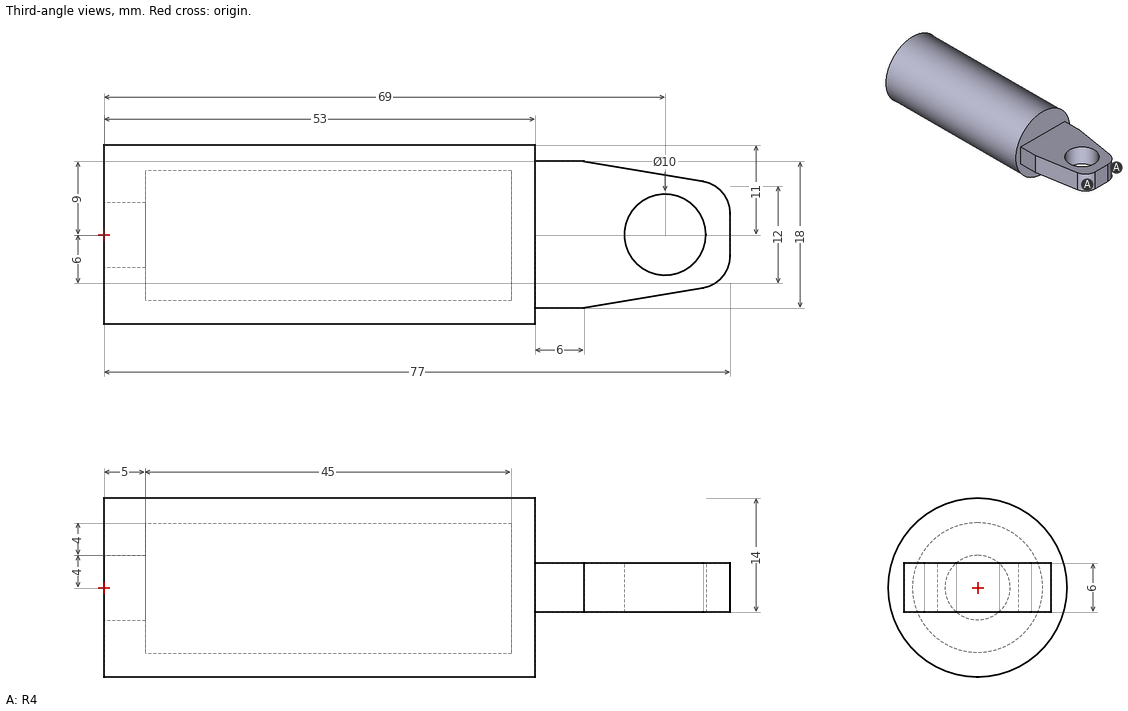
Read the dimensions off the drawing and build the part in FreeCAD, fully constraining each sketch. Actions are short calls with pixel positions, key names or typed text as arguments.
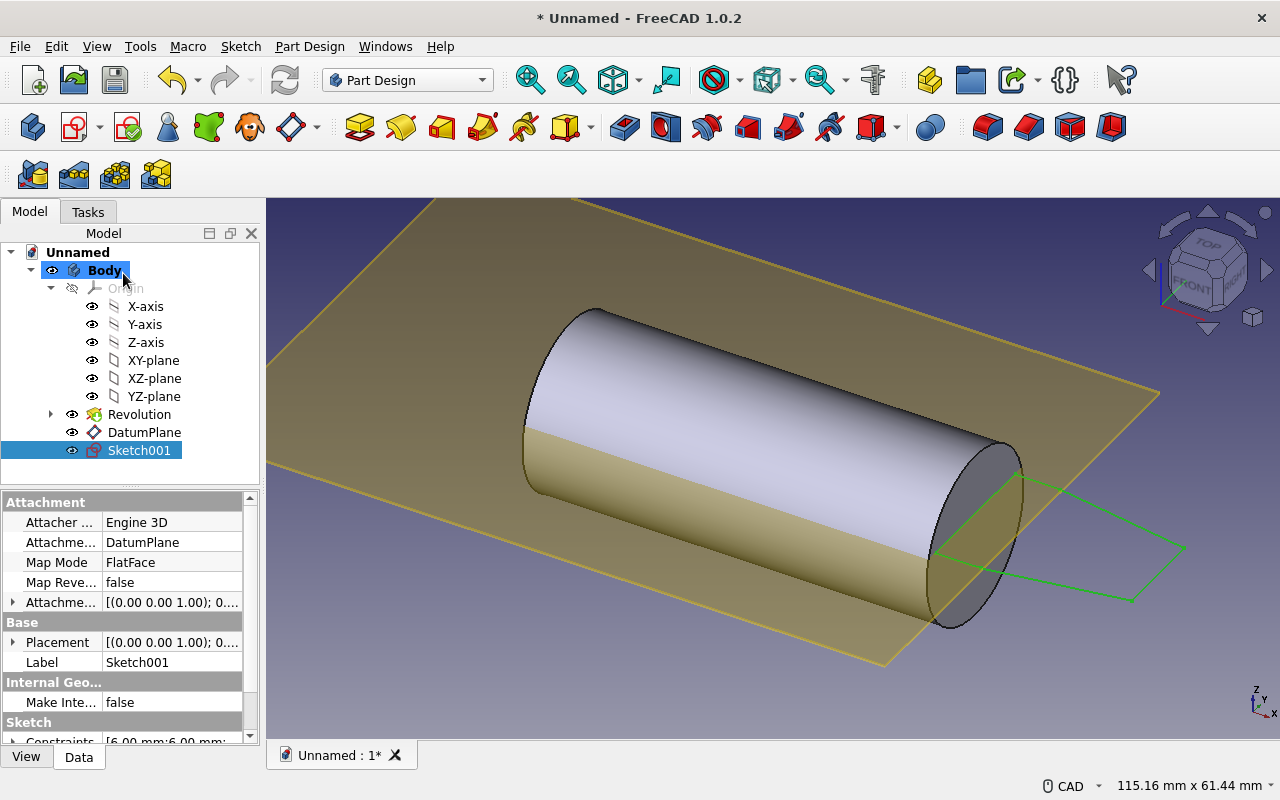
click(360, 128)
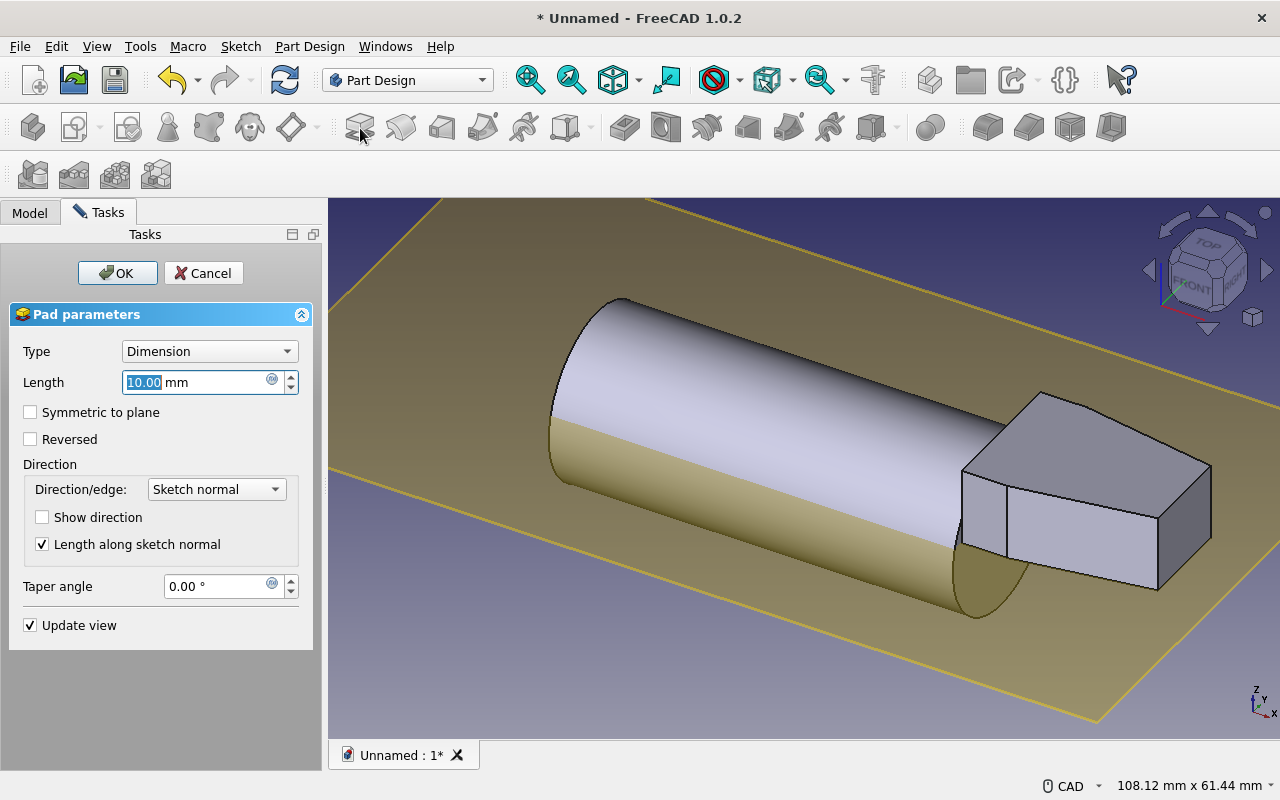
text(6)
key(Tab)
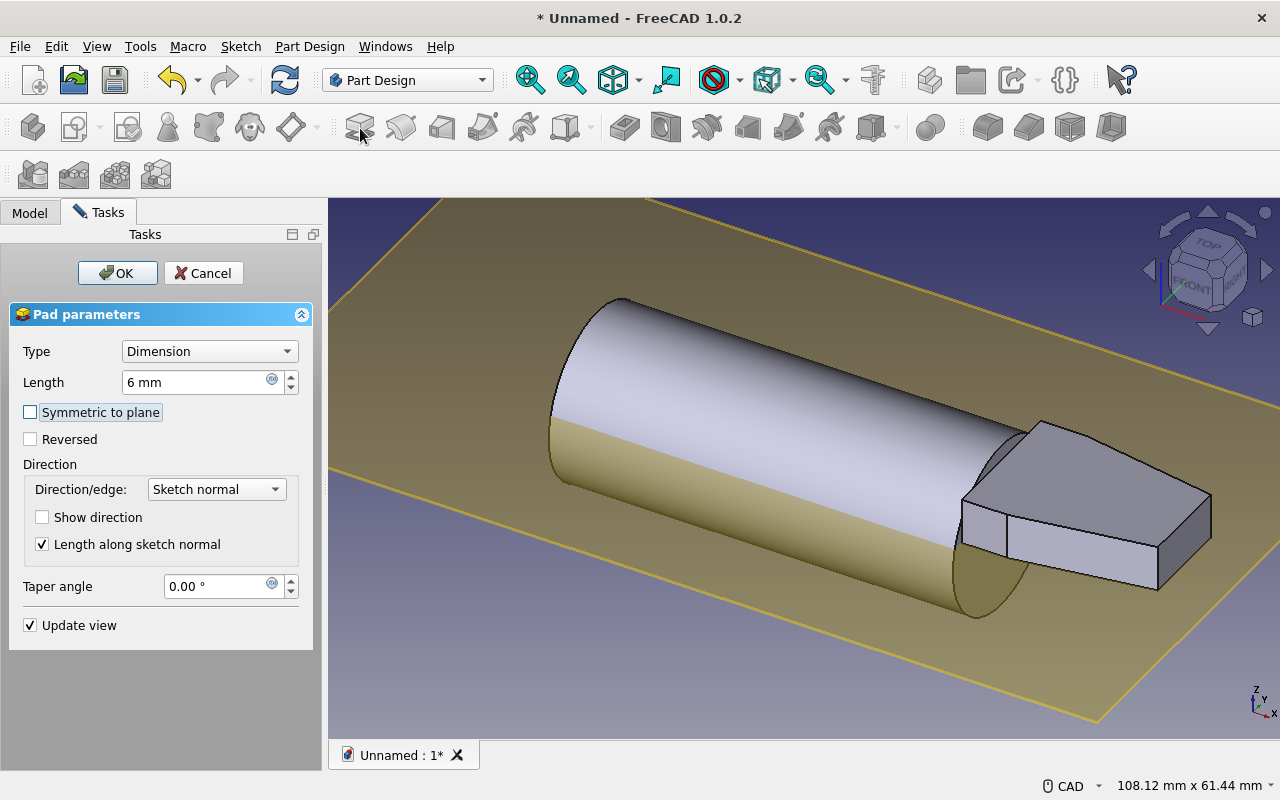
click(31, 439)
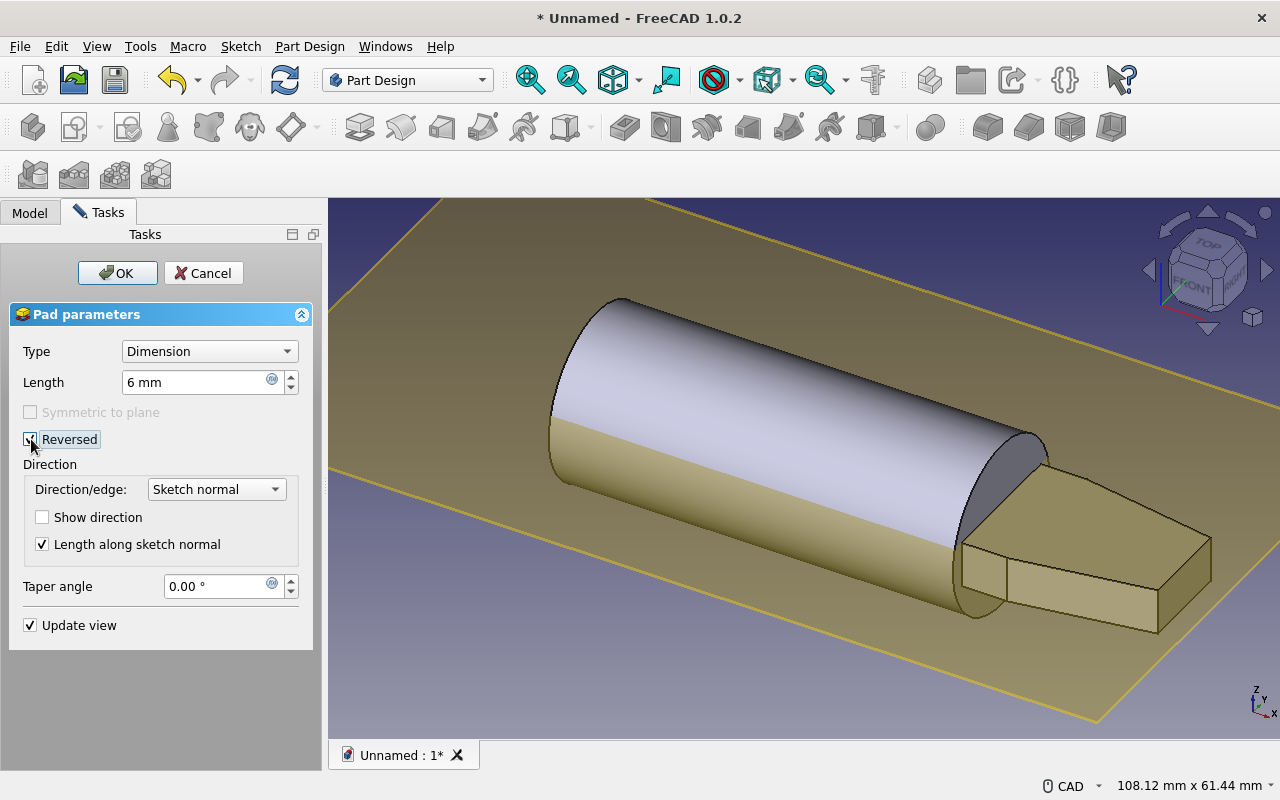
click(118, 273)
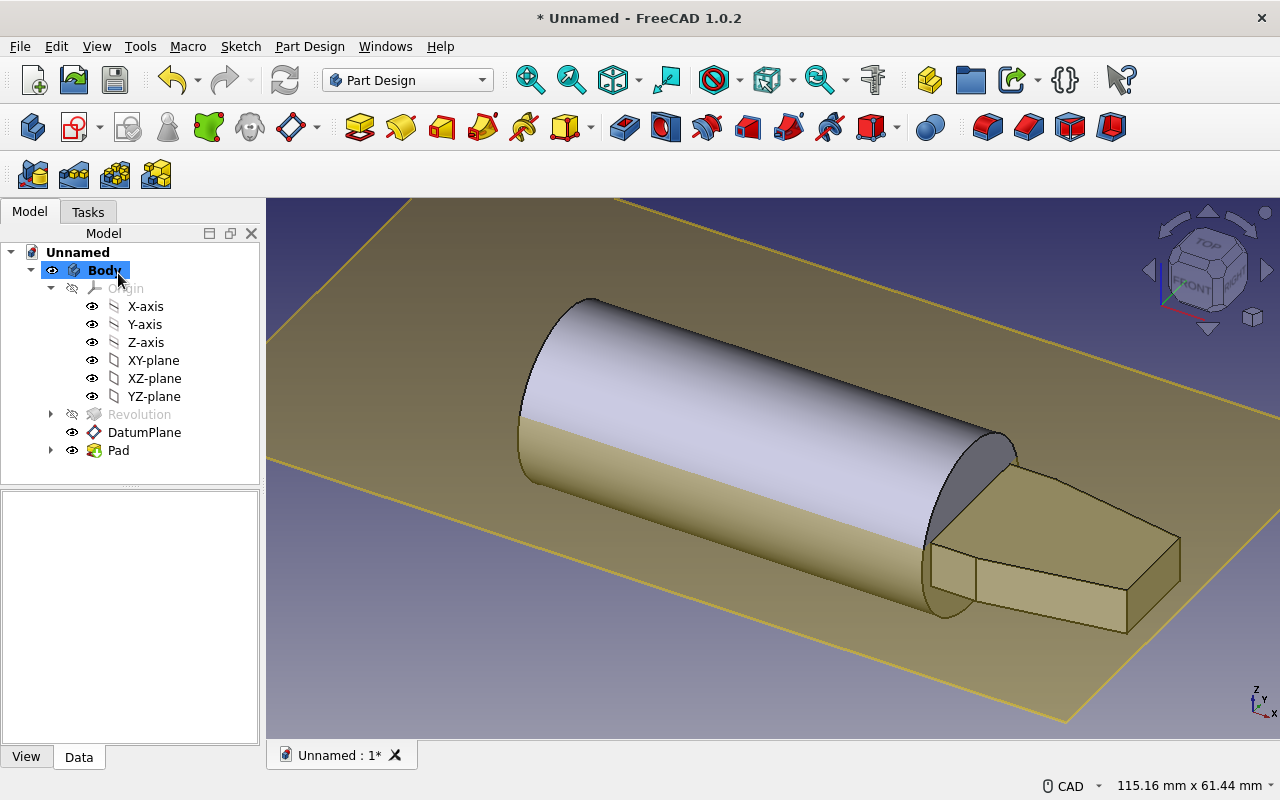
click(117, 432)
key(space)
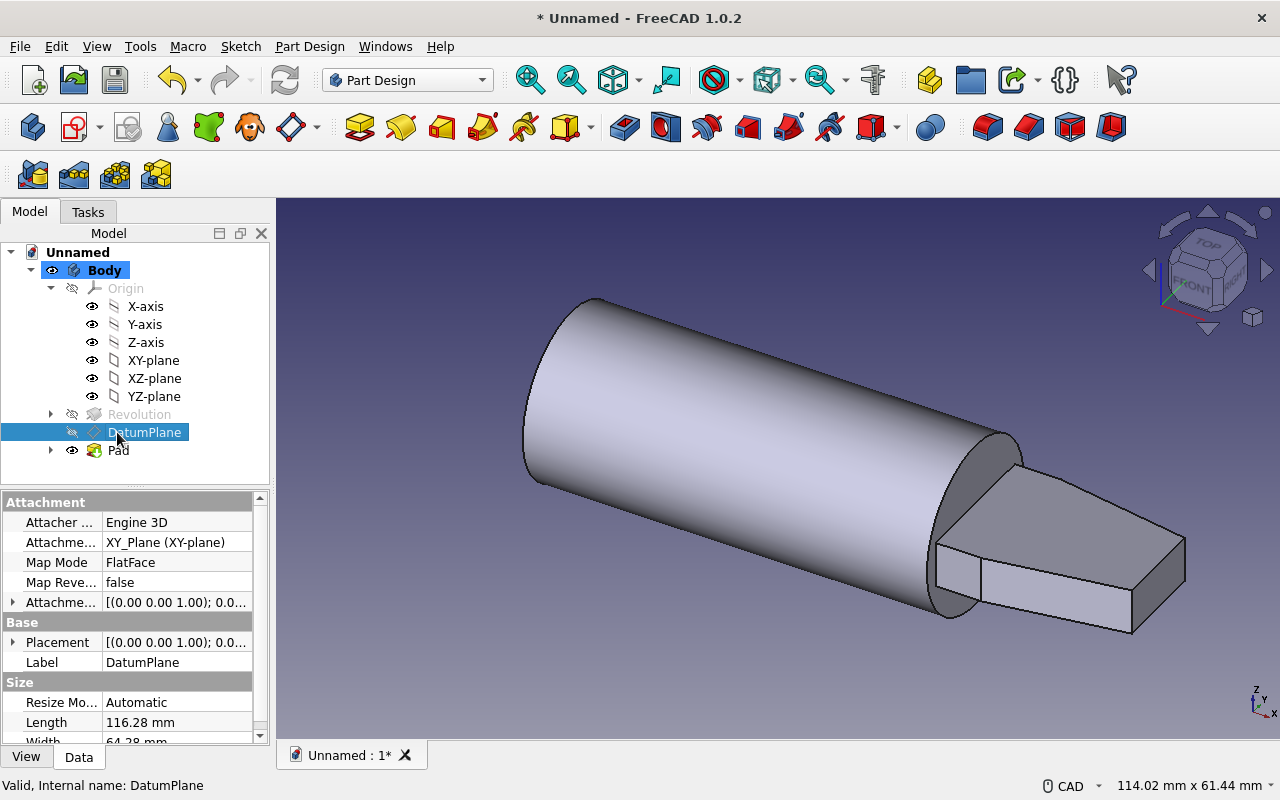
key(5)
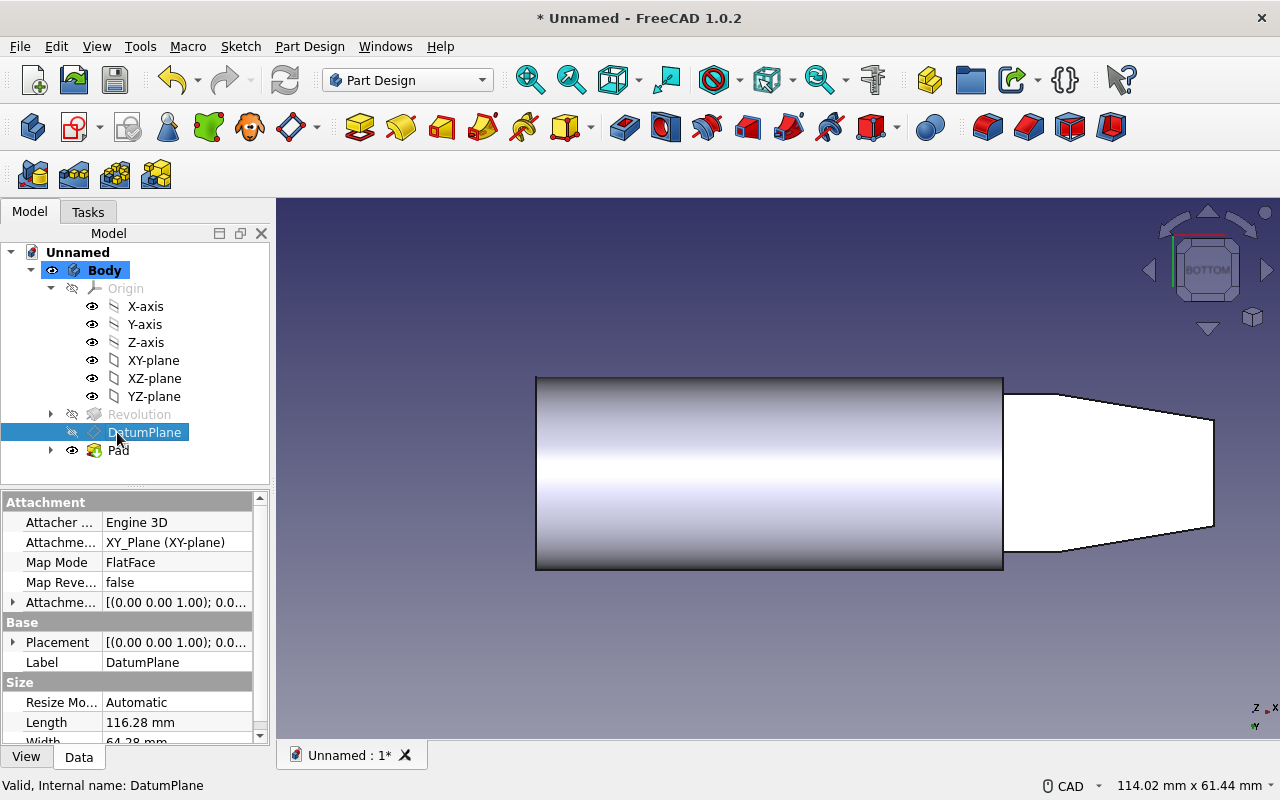
click(1079, 472)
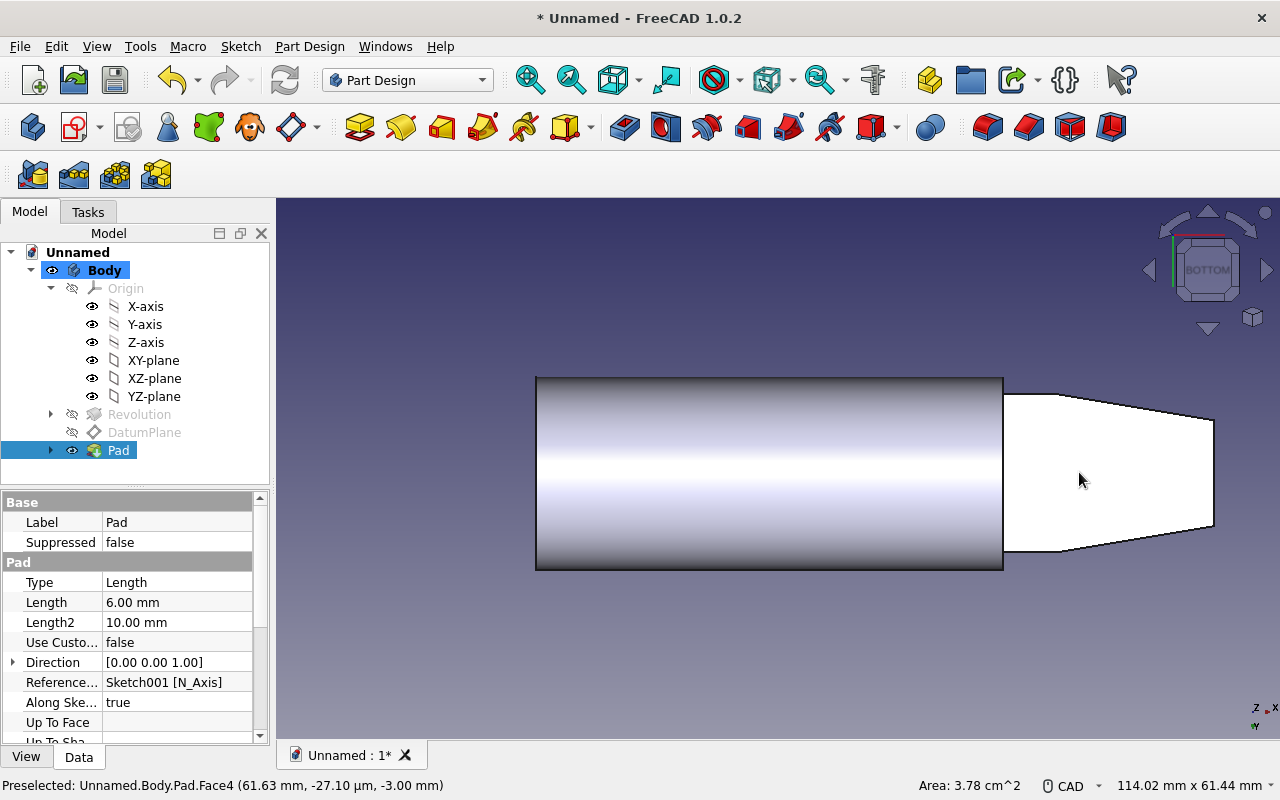
click(74, 128)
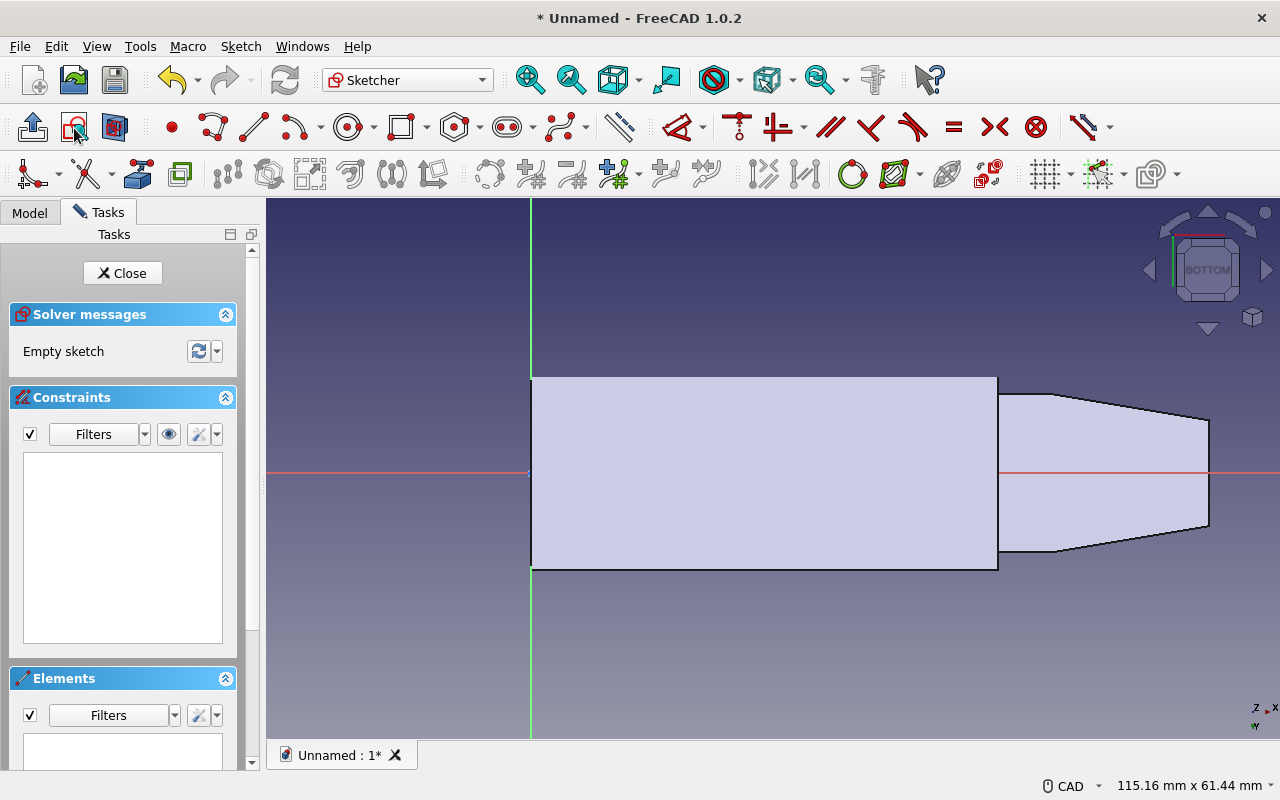
scroll(704, 468, down, 5)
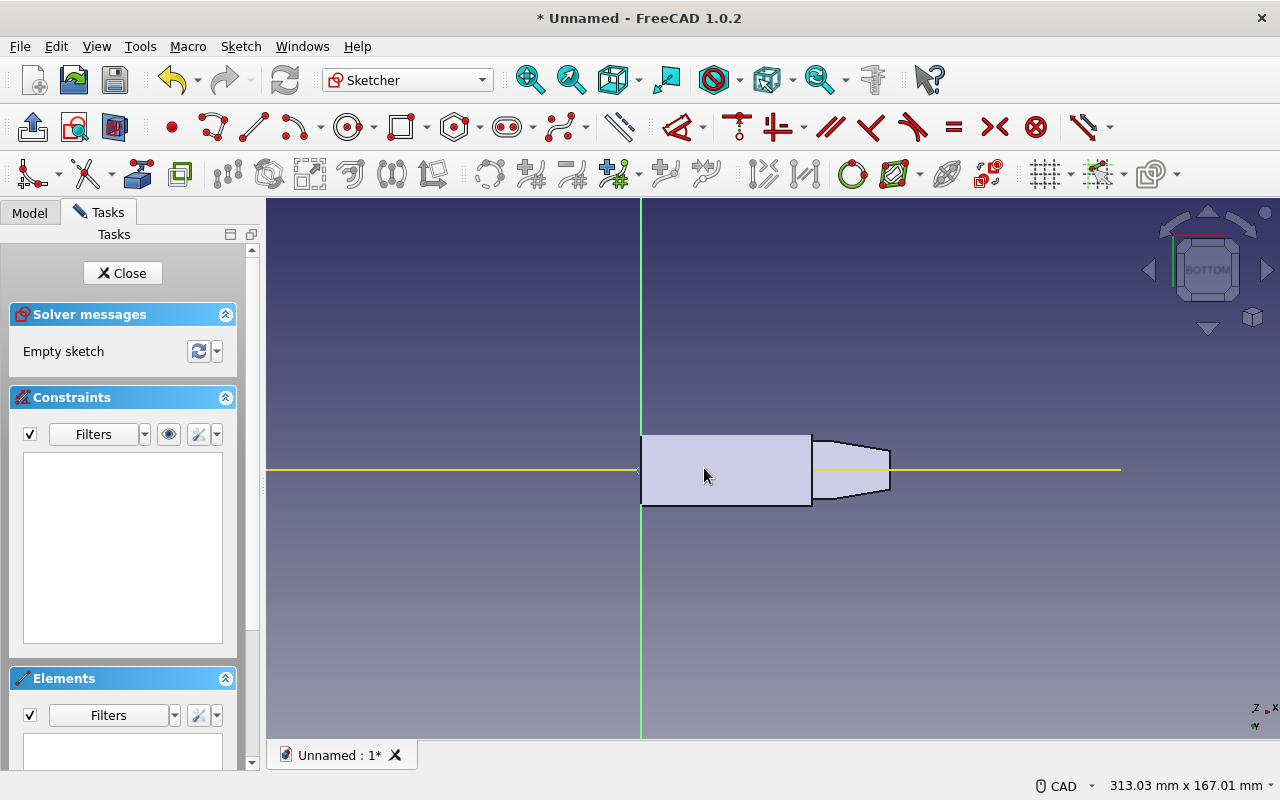
scroll(880, 470, up, 12)